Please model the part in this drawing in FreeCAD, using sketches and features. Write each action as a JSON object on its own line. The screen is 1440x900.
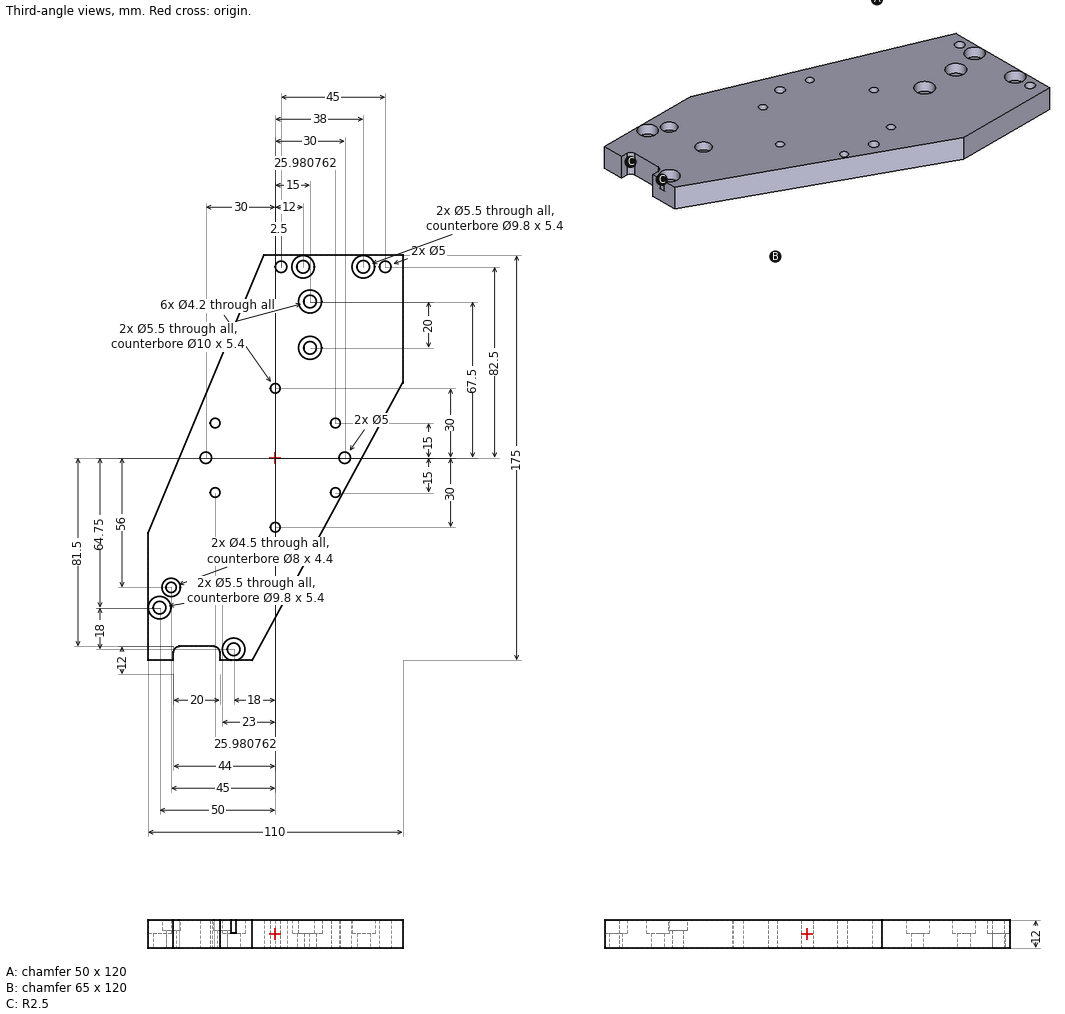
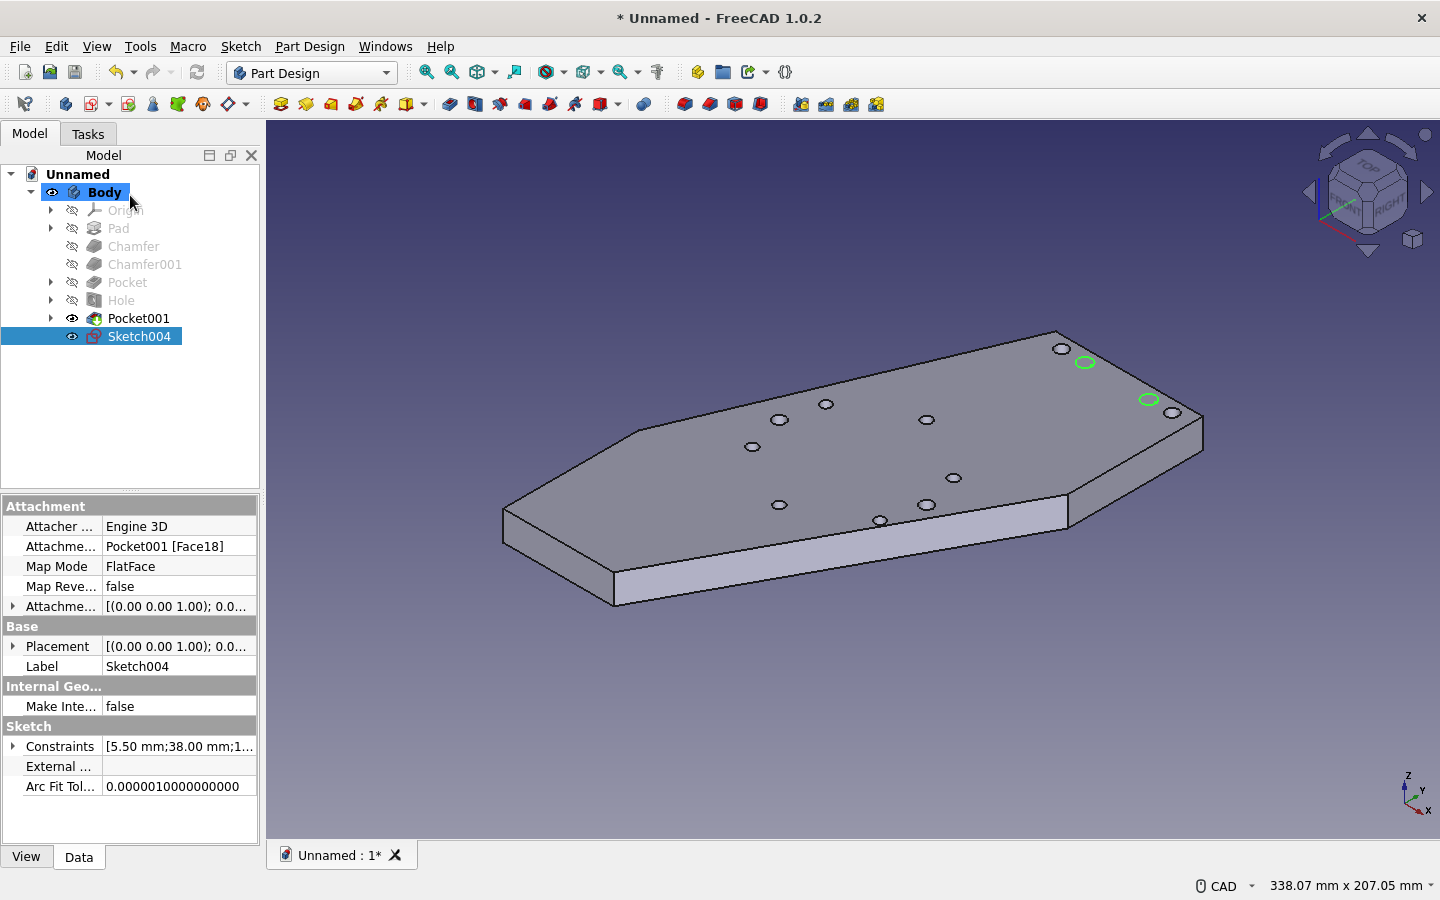
{"action": "left_click", "coordinate": [475, 104]}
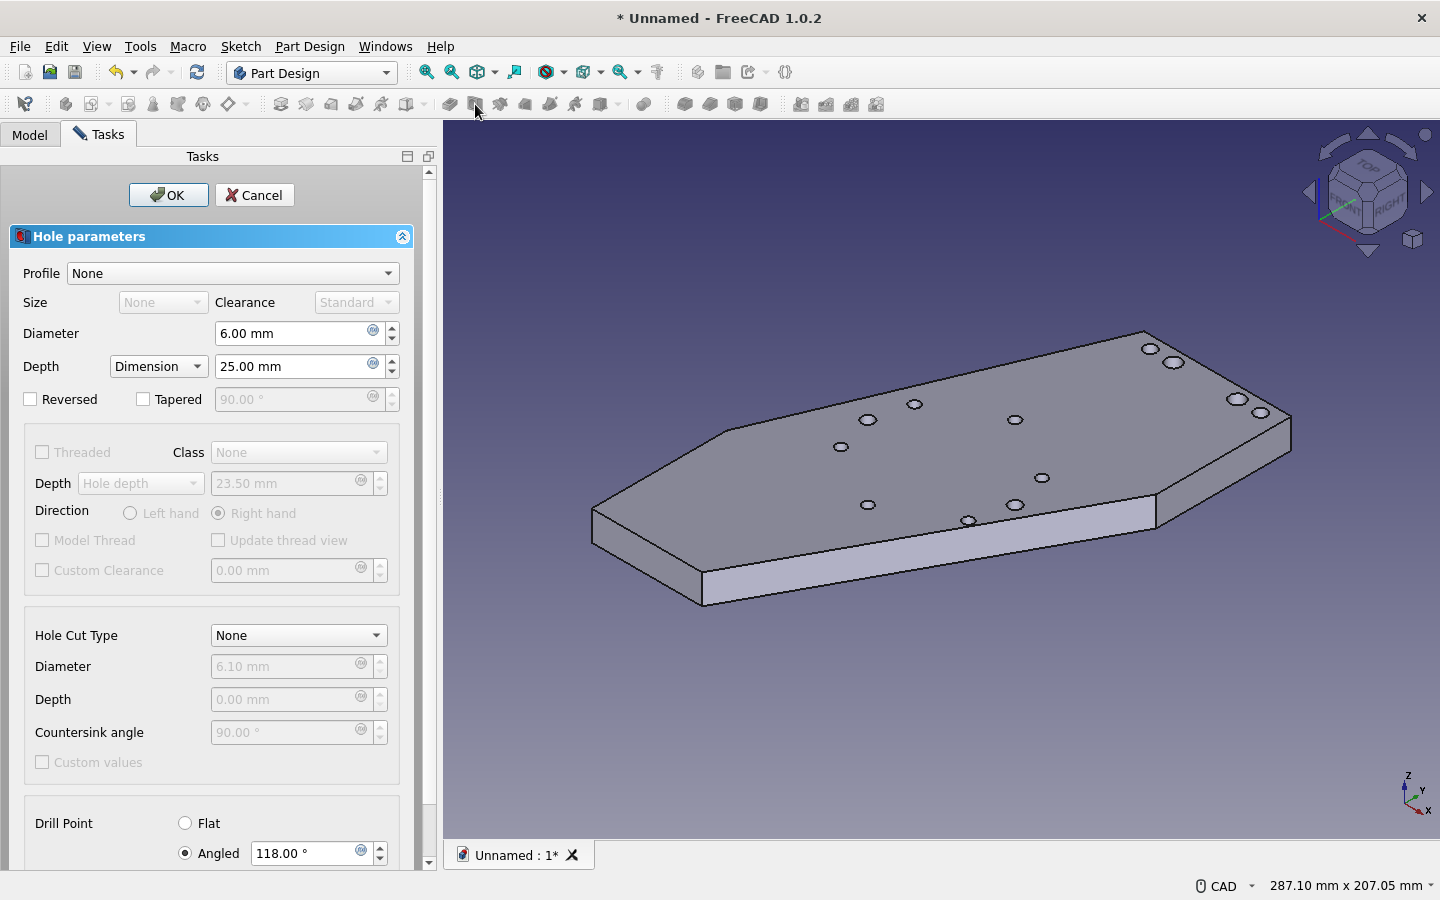
{"action": "triple_click", "coordinate": [300, 334]}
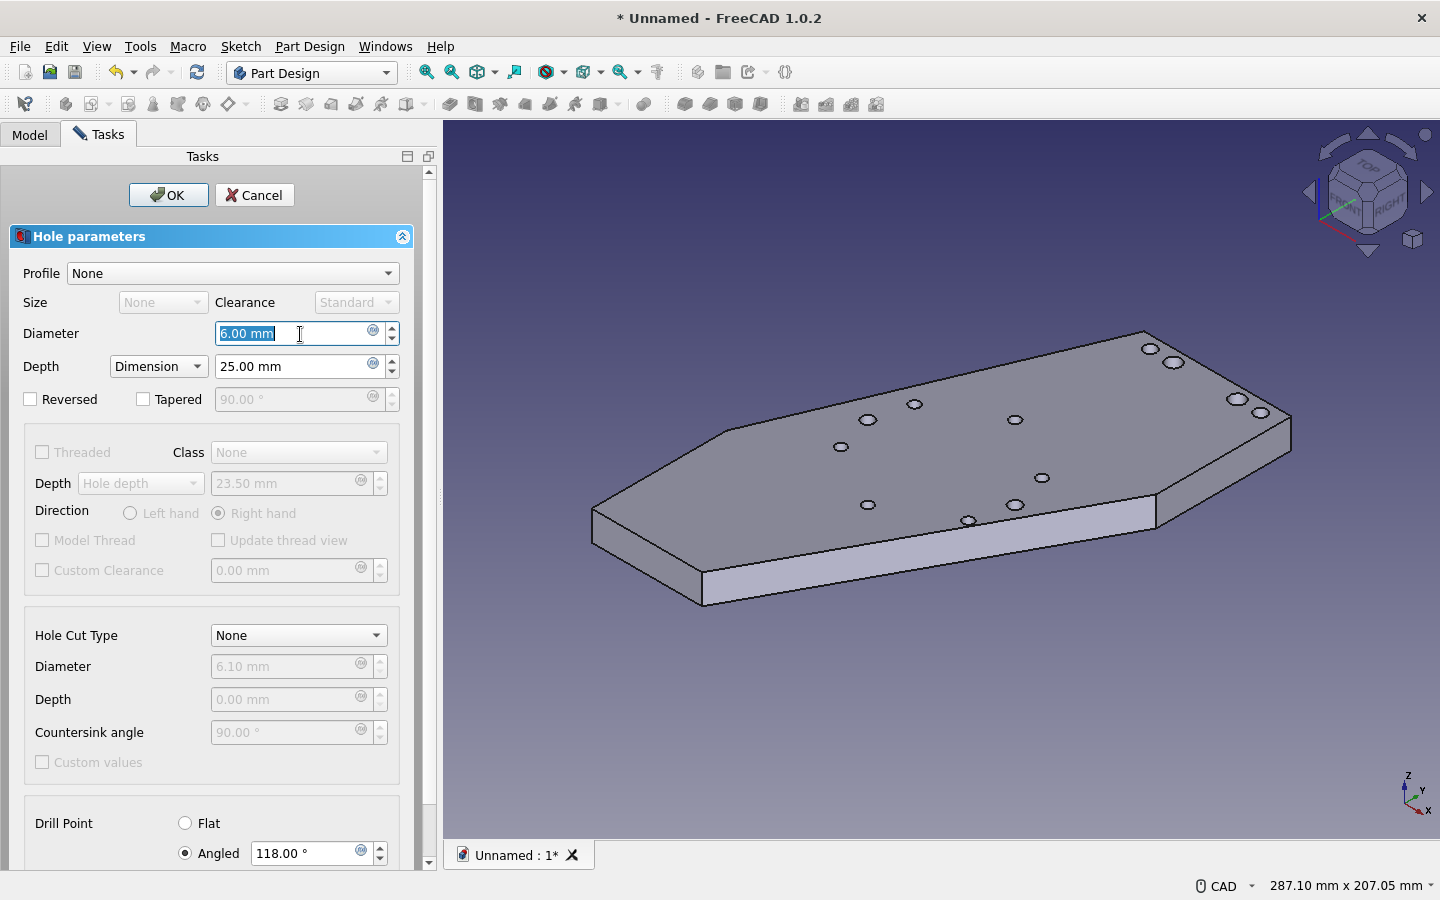
{"action": "type", "text": "5.5"}
{"action": "key", "text": "Tab"}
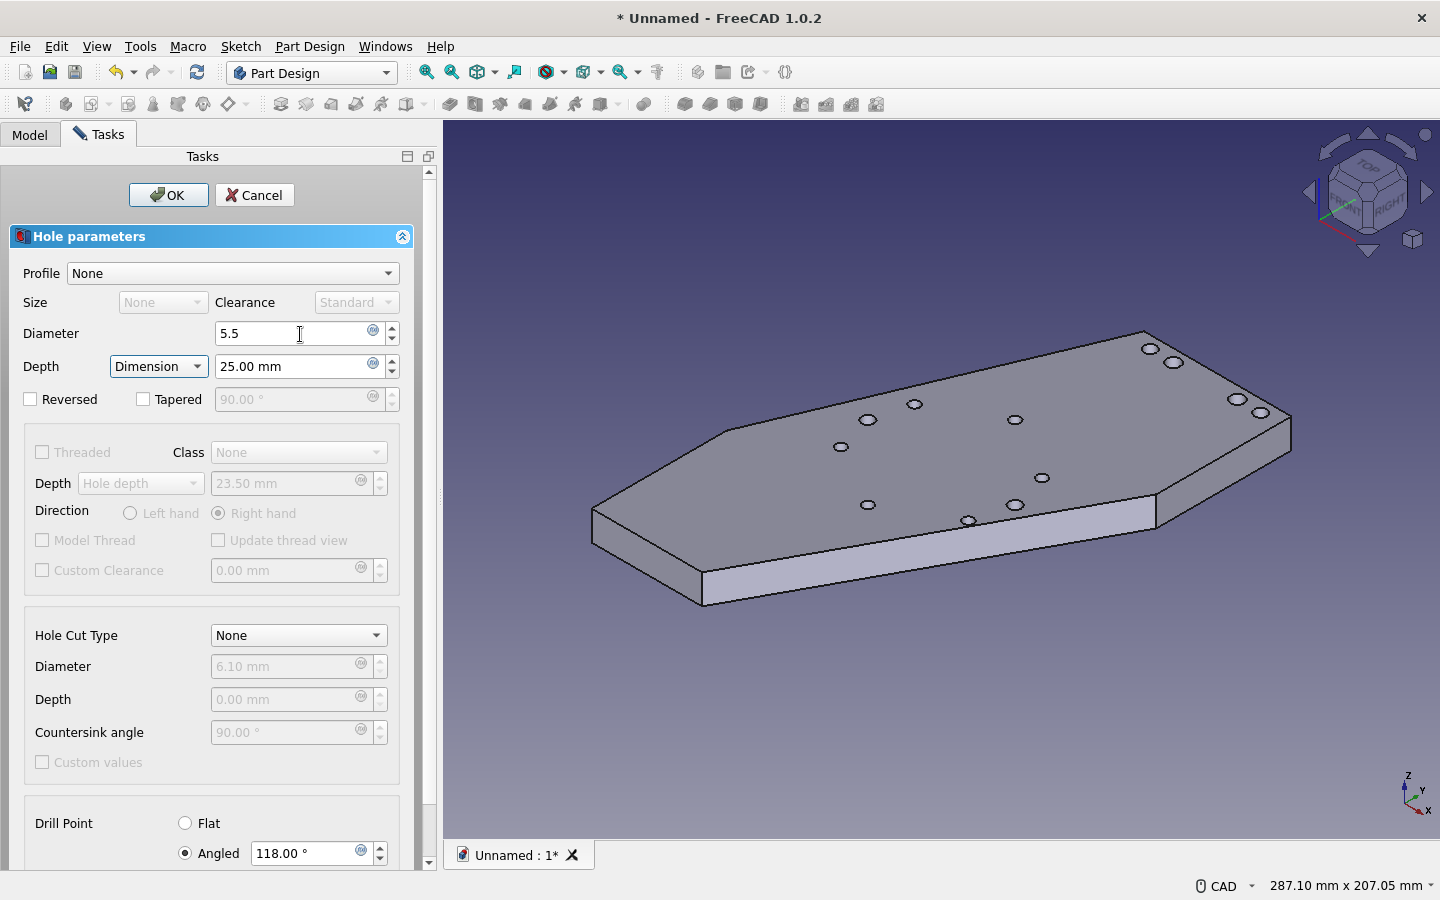
{"action": "left_click", "coordinate": [160, 366]}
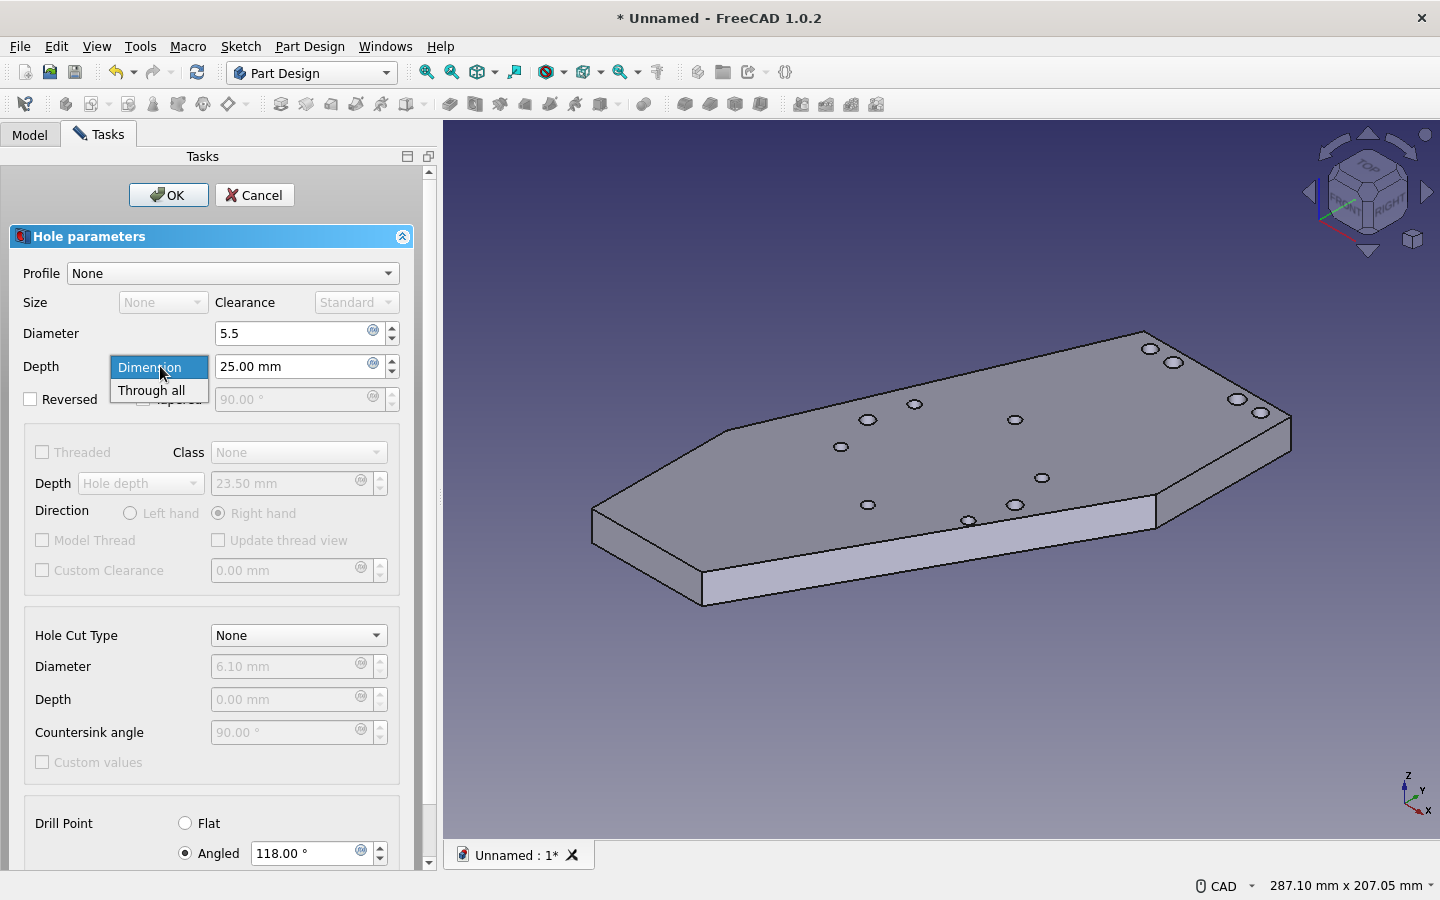
{"action": "left_click", "coordinate": [158, 390]}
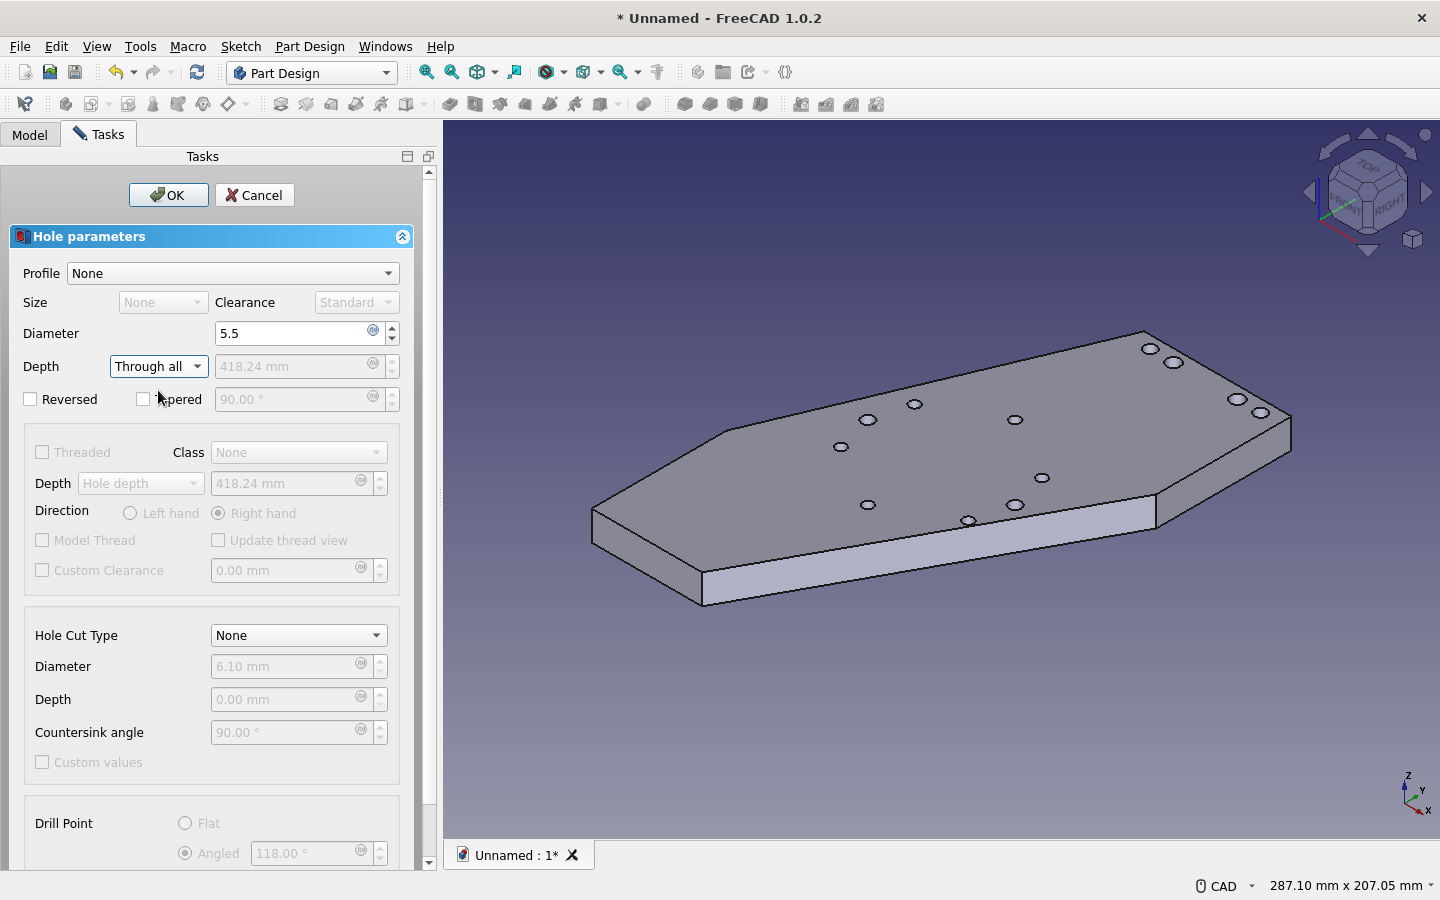
{"action": "left_click", "coordinate": [300, 636]}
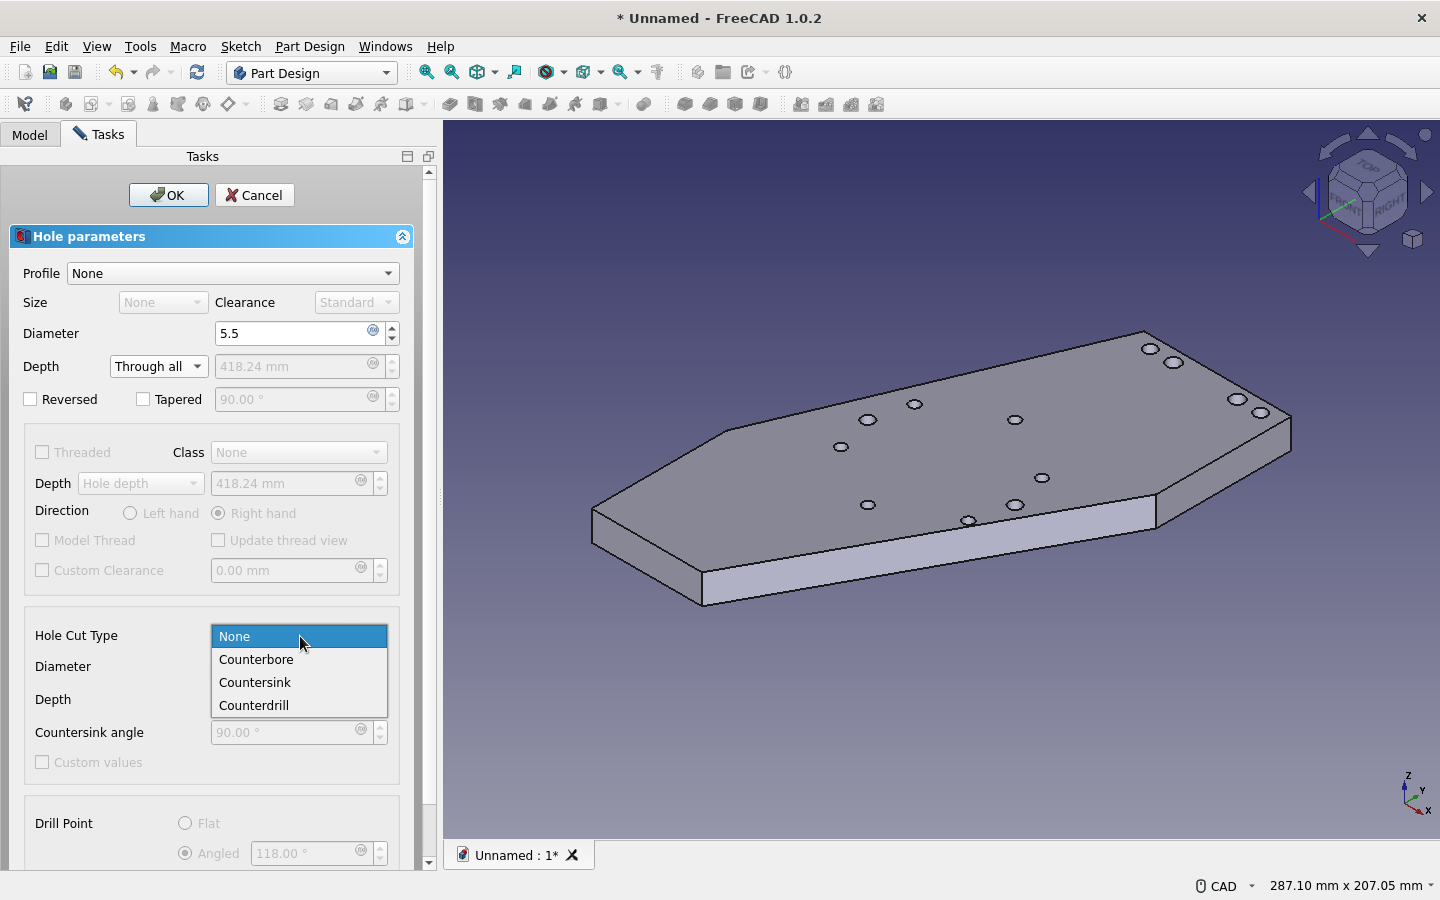
{"action": "left_click", "coordinate": [298, 660]}